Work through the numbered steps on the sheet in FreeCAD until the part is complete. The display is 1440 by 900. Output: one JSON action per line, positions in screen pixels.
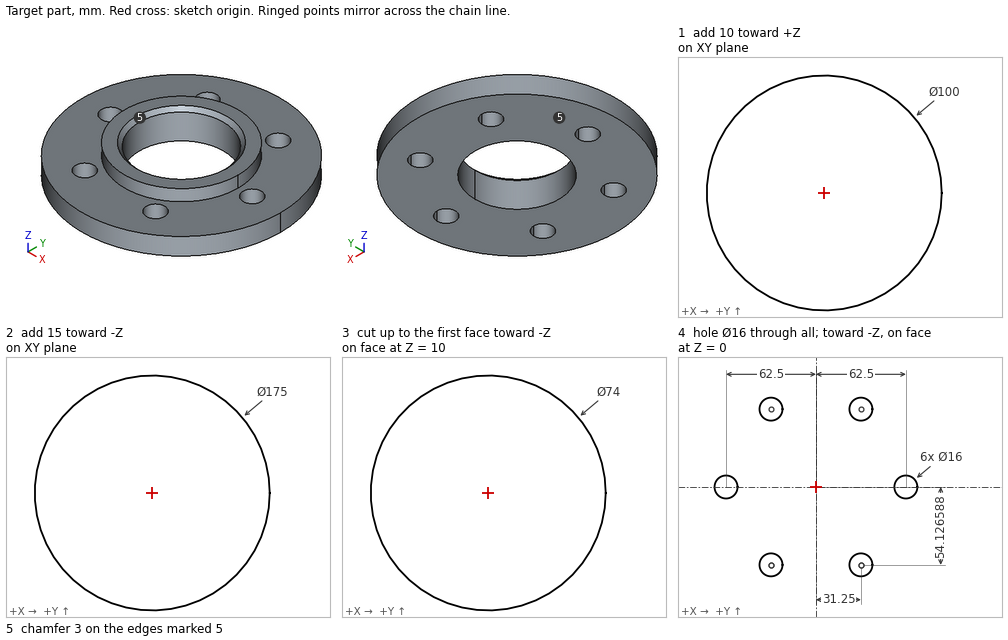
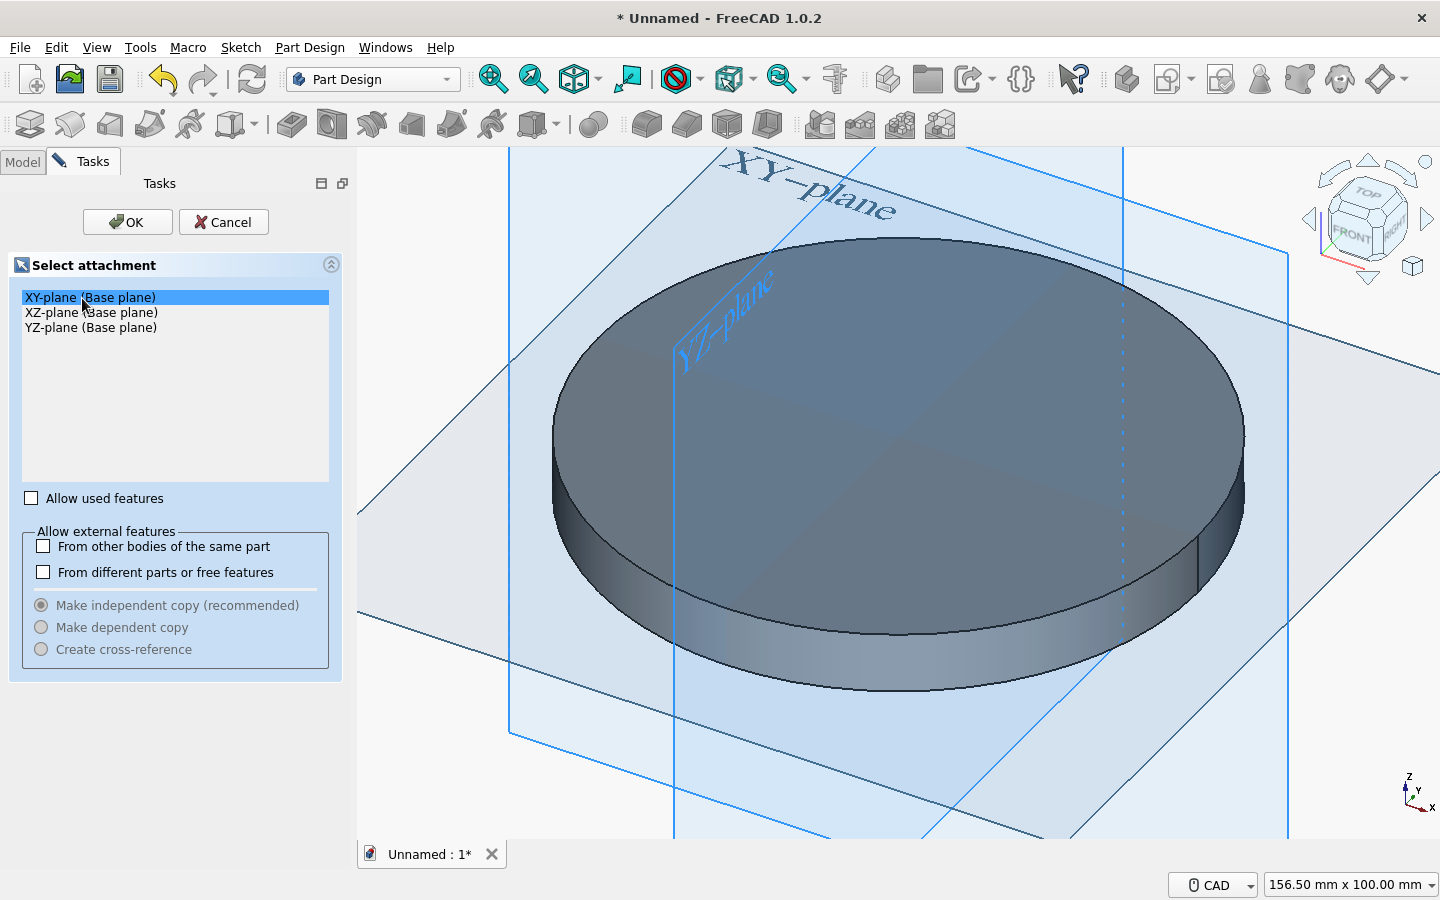
{"action": "left_click", "coordinate": [128, 222]}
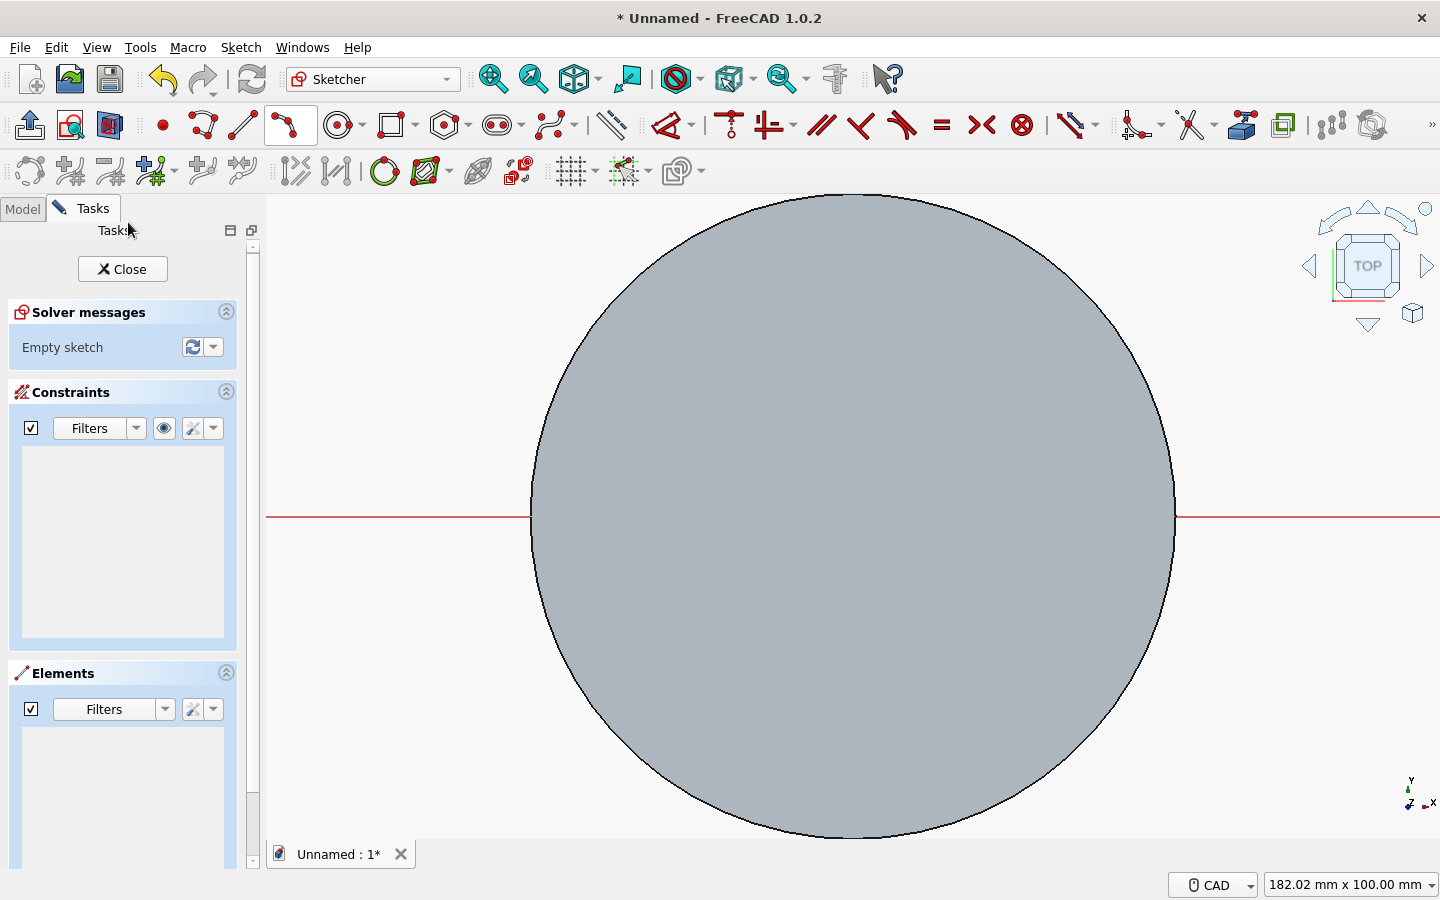
{"action": "left_click", "coordinate": [110, 126]}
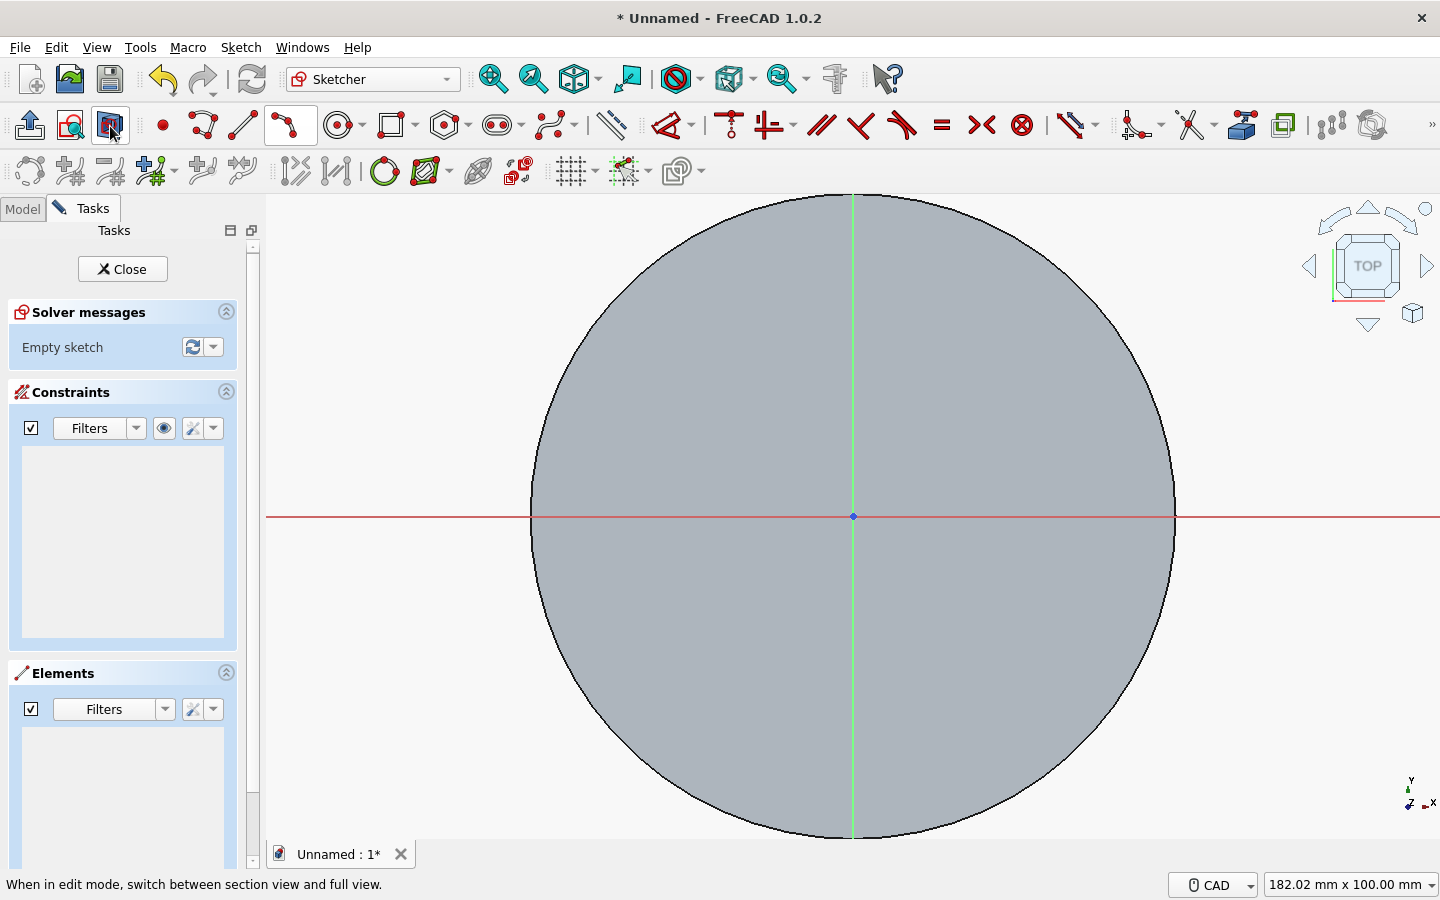
{"action": "scroll", "coordinate": [745, 516], "scroll_direction": "down", "scroll_amount": 5}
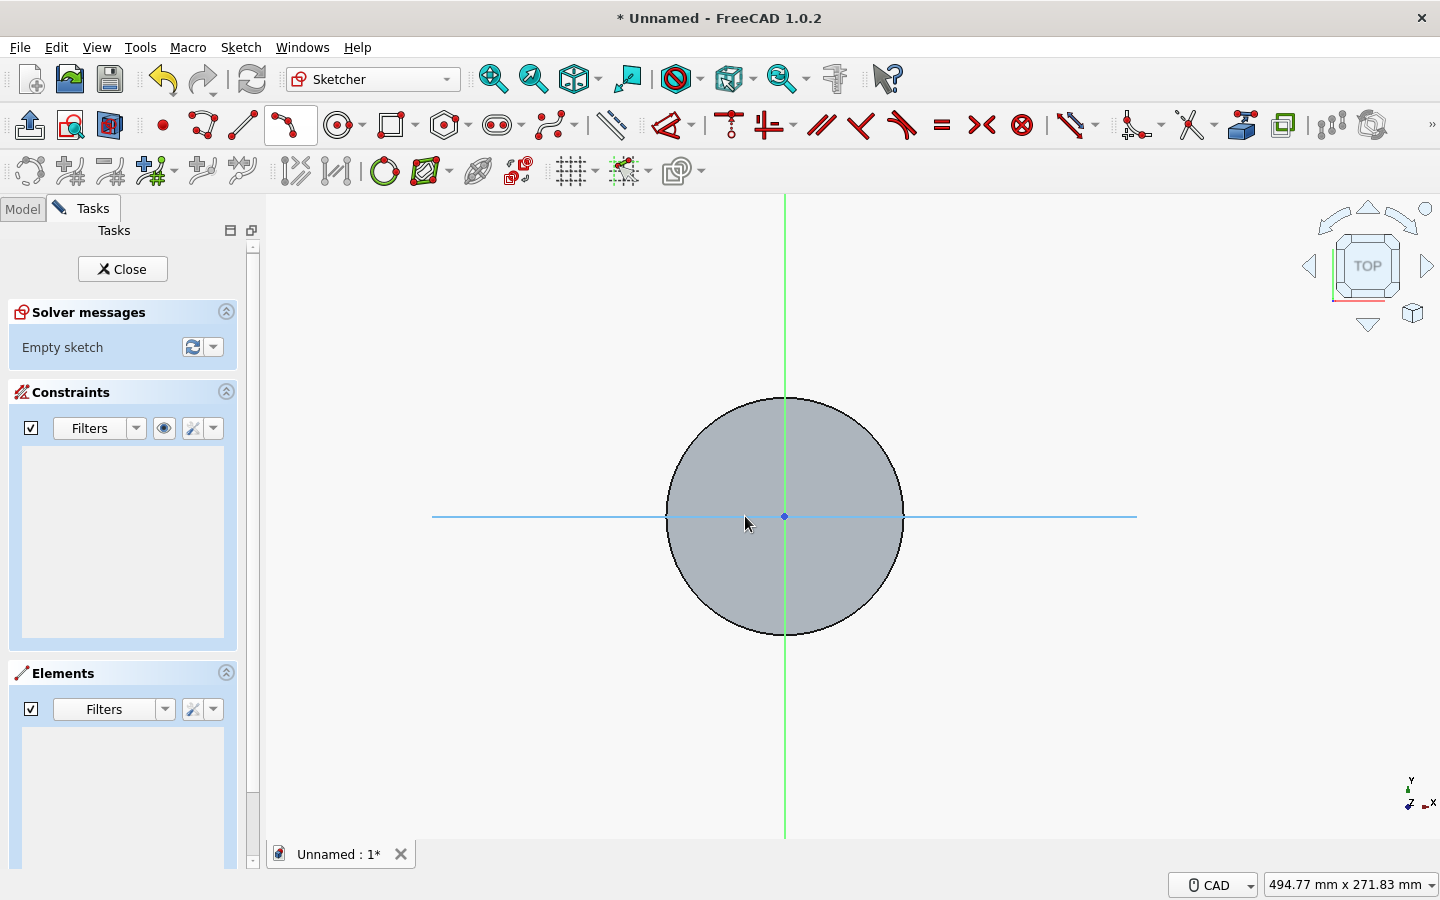
{"action": "left_click", "coordinate": [338, 126]}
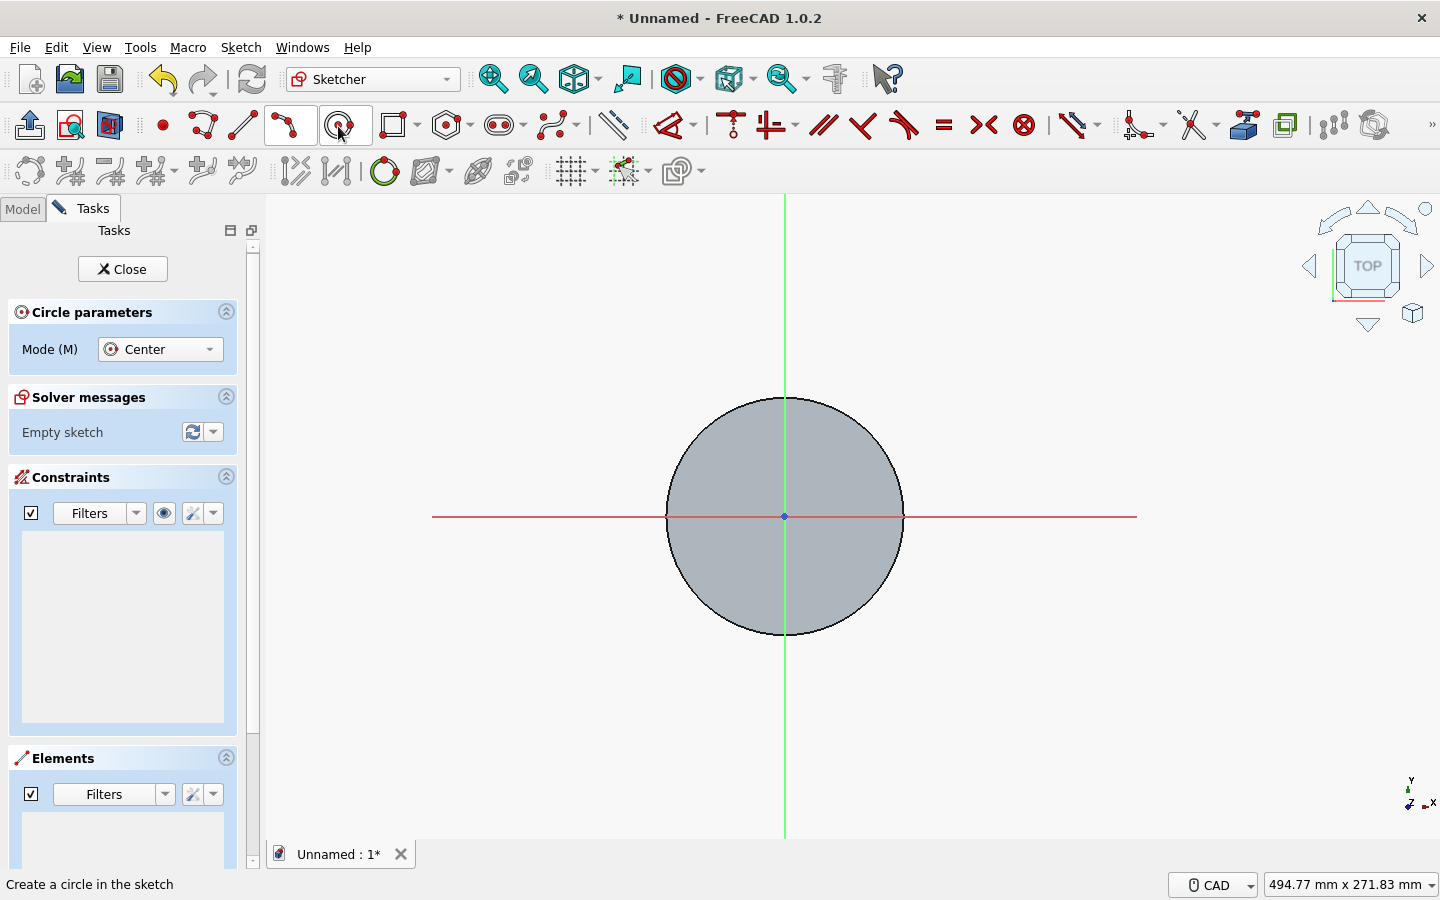
{"action": "left_click", "coordinate": [785, 516]}
{"action": "left_click", "coordinate": [932, 370]}
{"action": "key", "text": "Escape"}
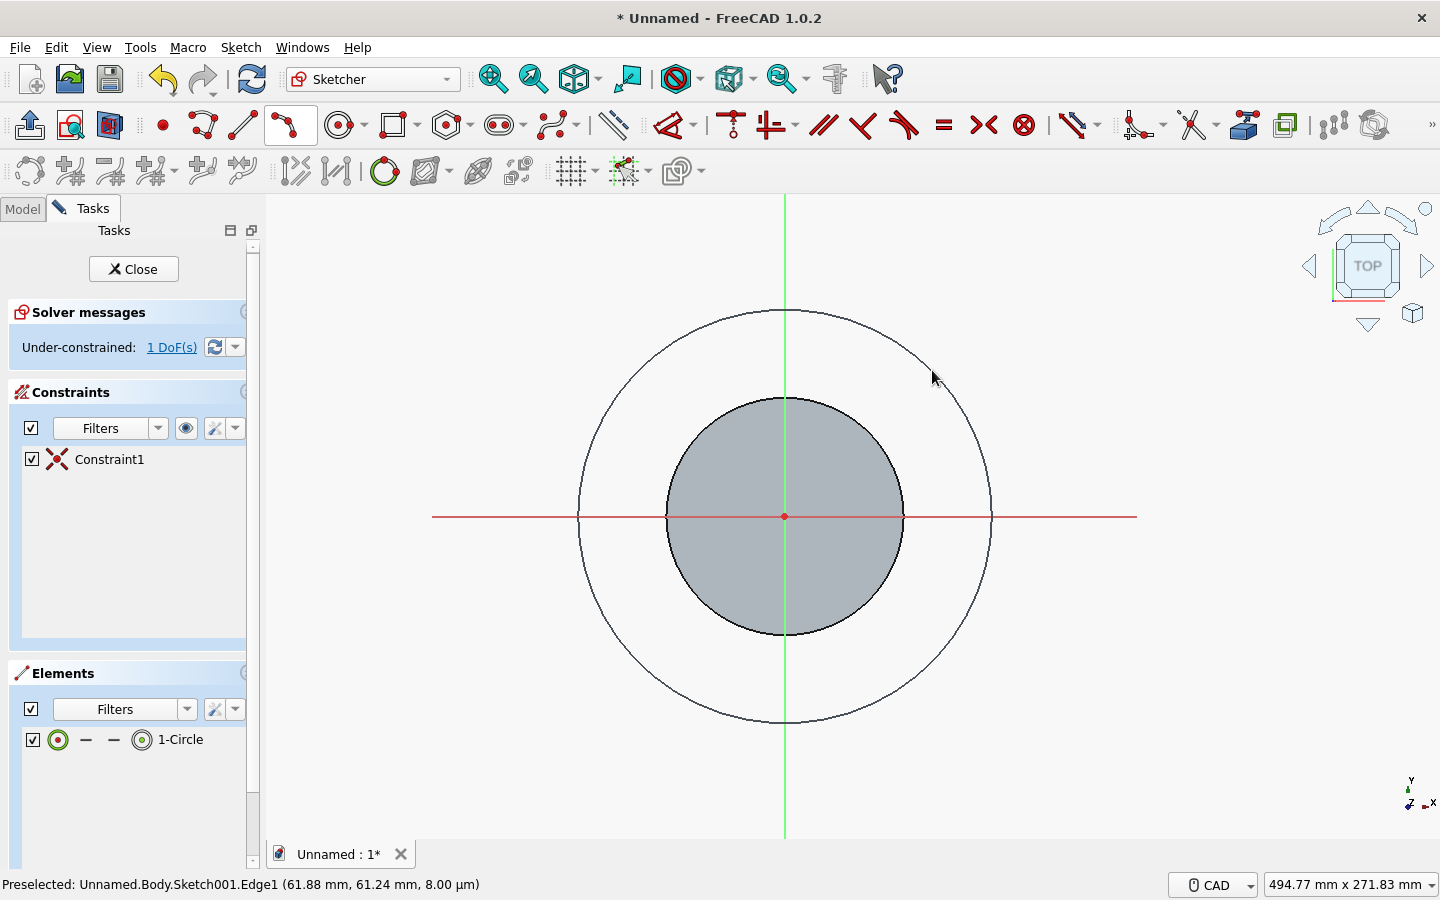
{"action": "left_click", "coordinate": [668, 126]}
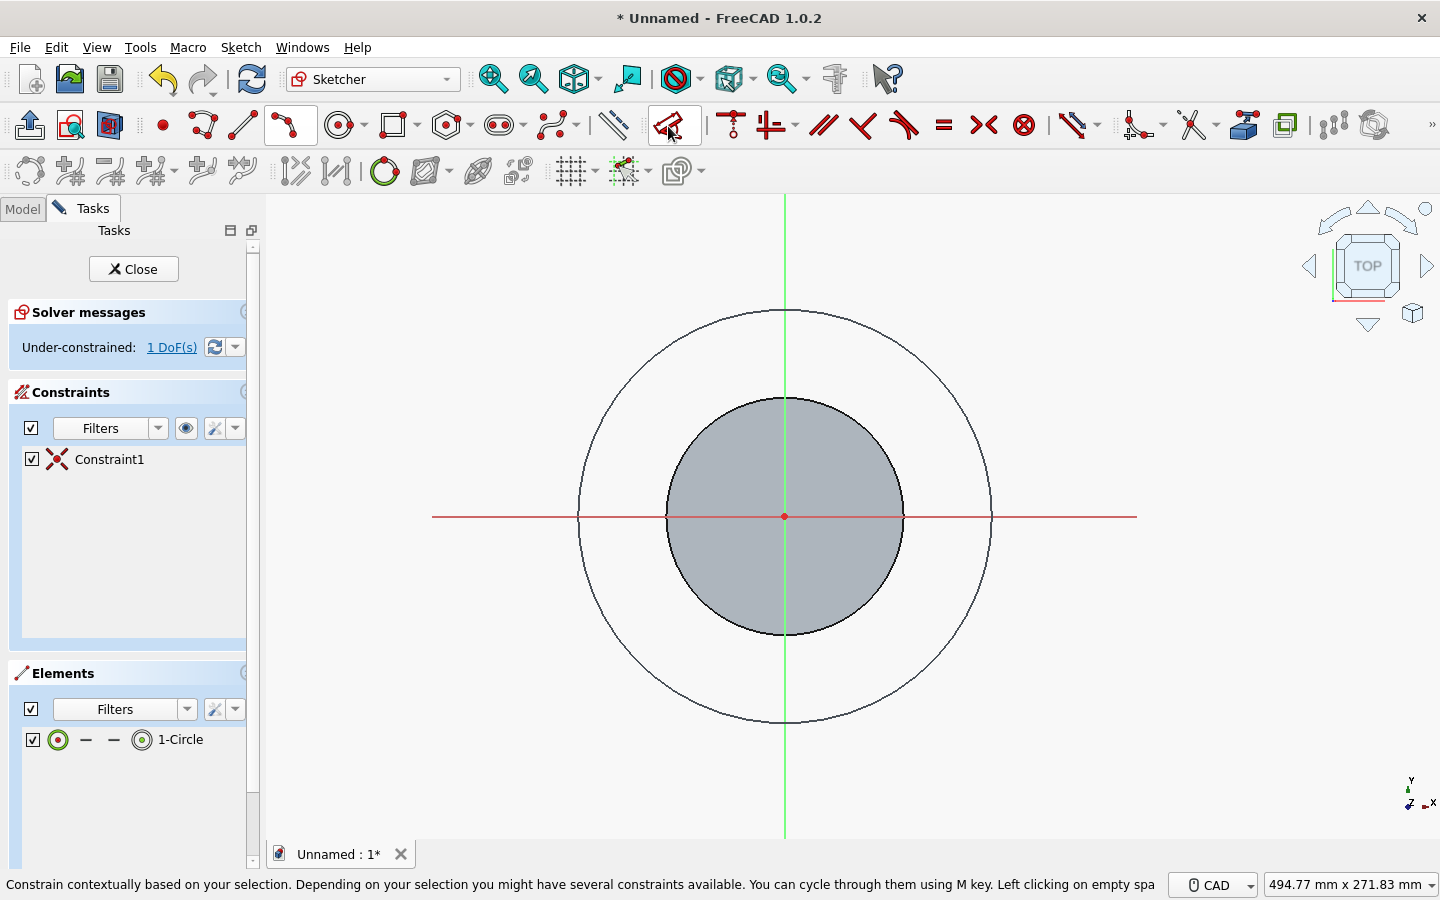
{"action": "left_click", "coordinate": [931, 370]}
{"action": "left_click", "coordinate": [954, 347]}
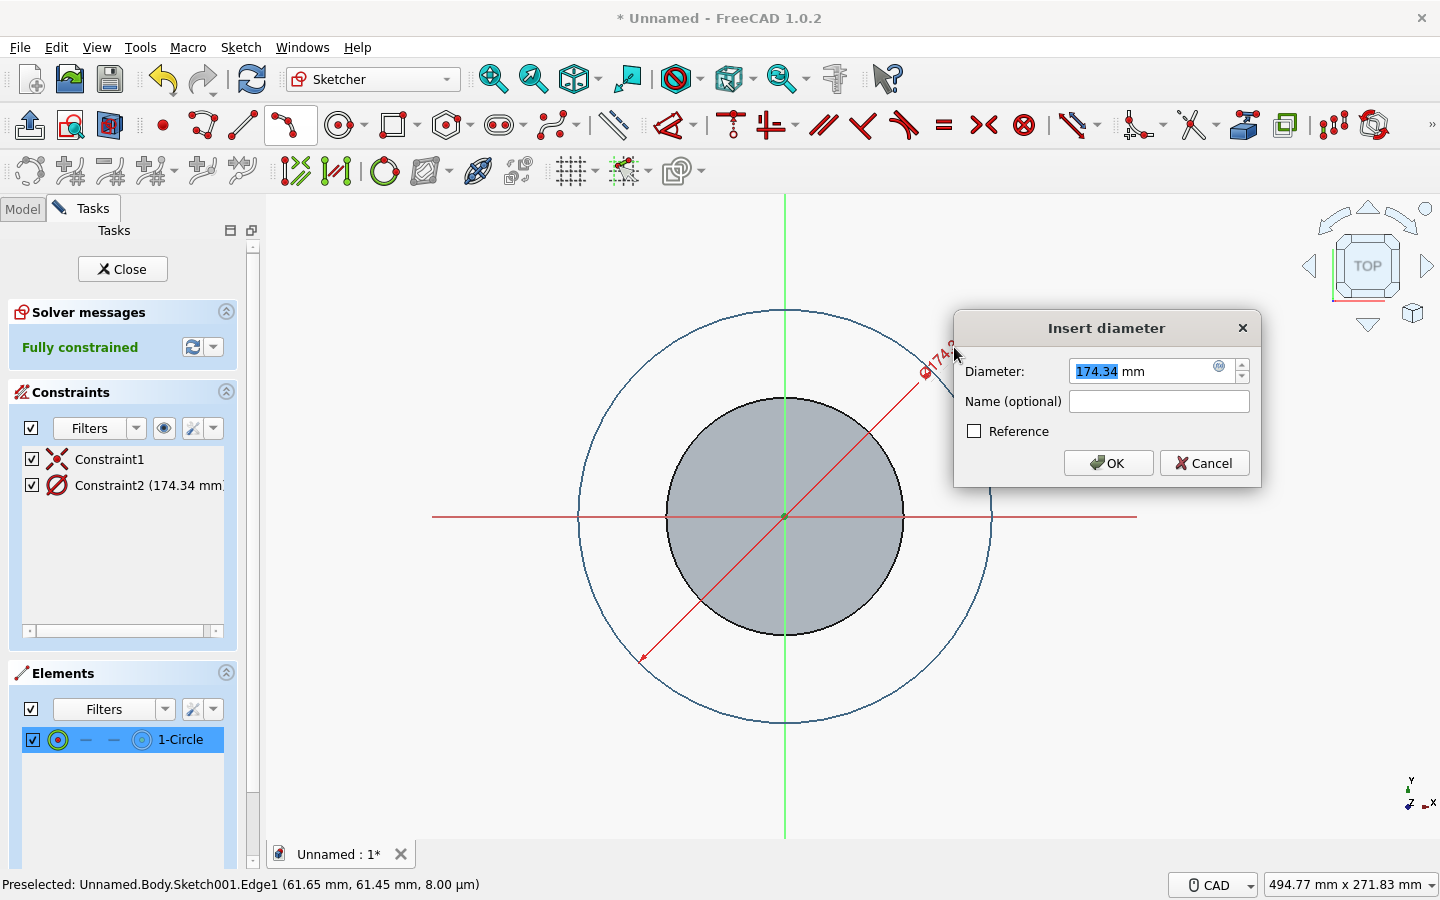
{"action": "type", "text": "175"}
{"action": "key", "text": "Return"}
{"action": "key", "text": "Escape"}